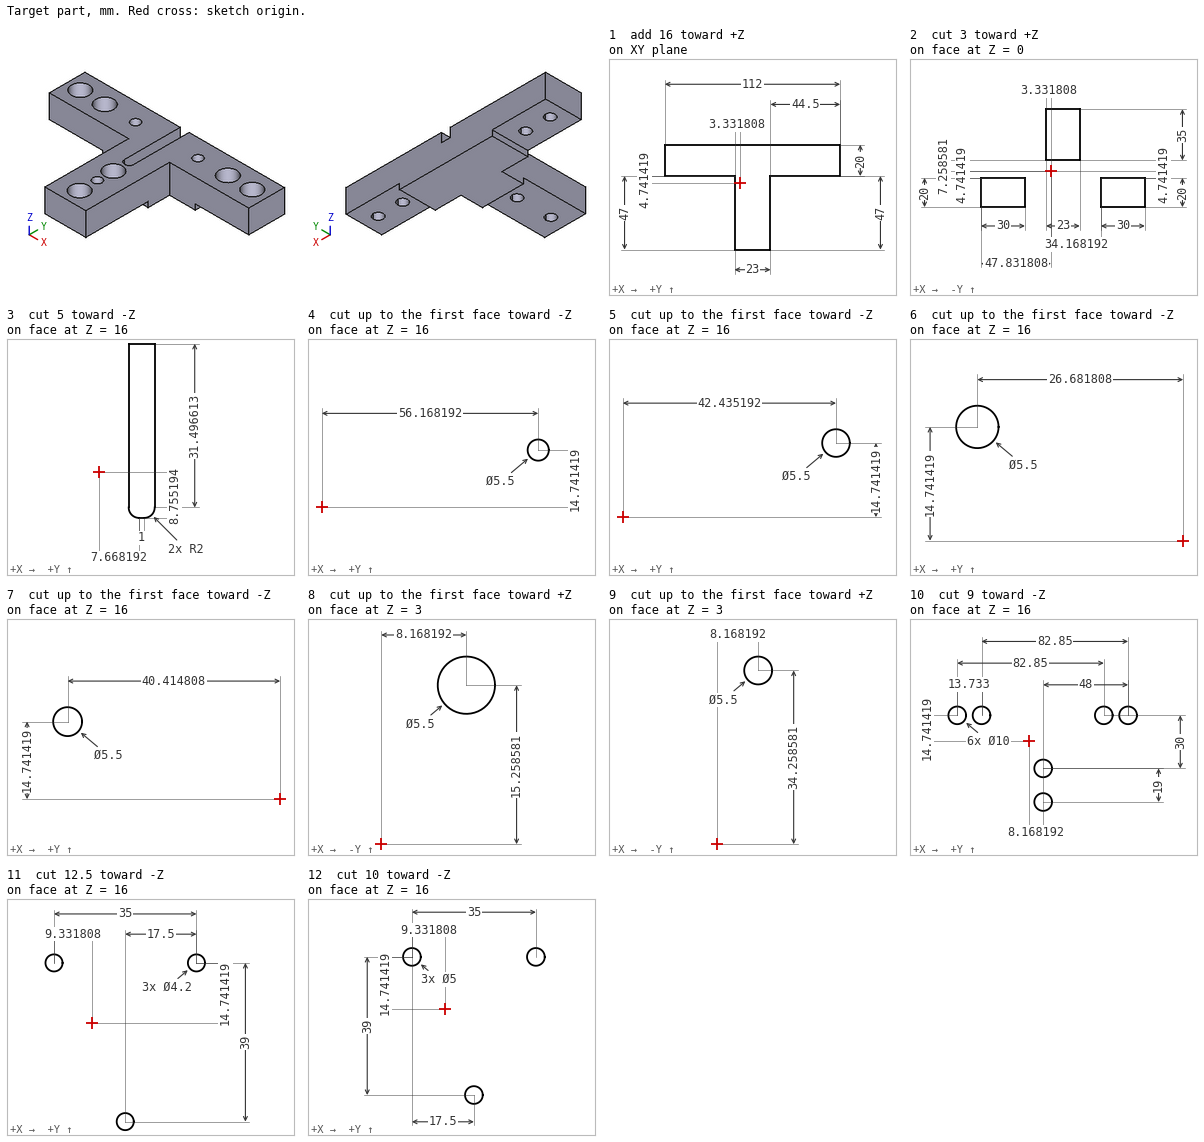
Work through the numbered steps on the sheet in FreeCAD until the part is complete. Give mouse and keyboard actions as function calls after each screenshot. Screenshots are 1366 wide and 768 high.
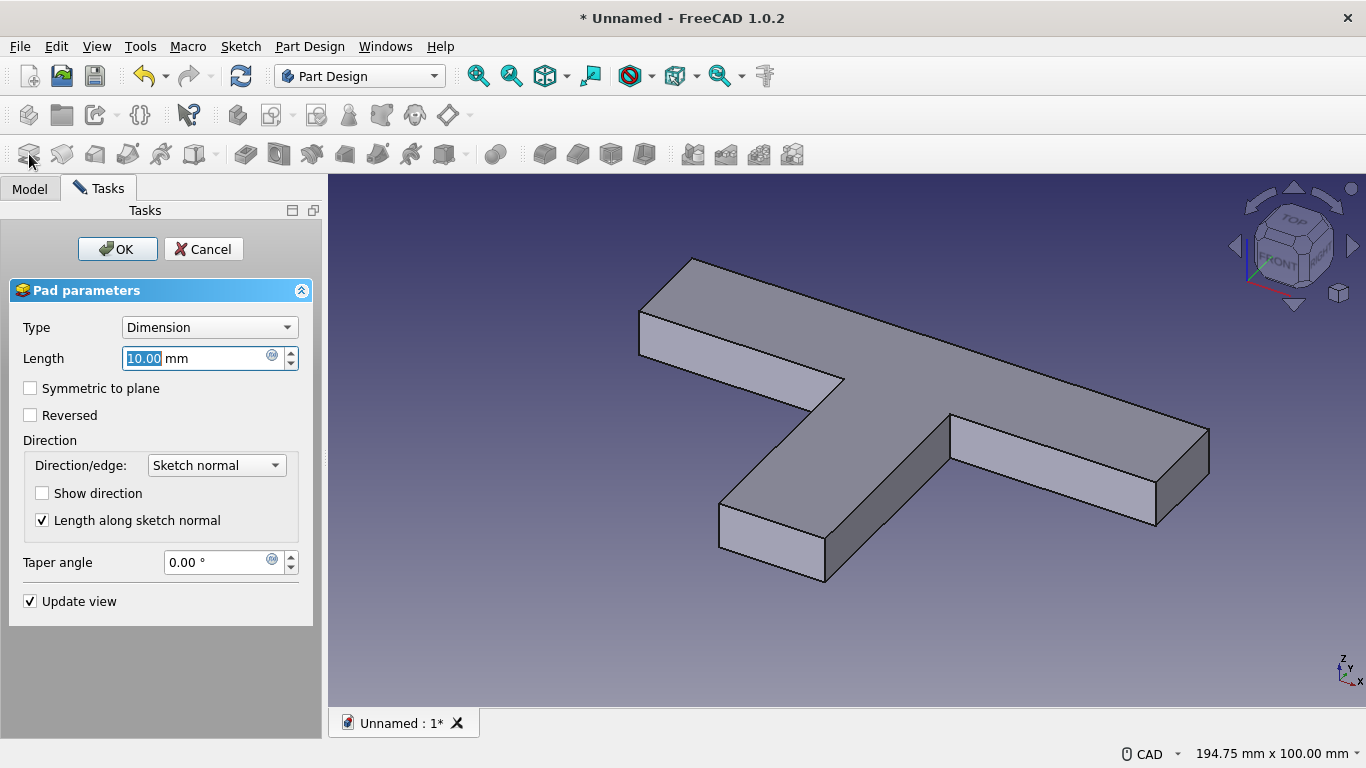
text(16)
key(Tab)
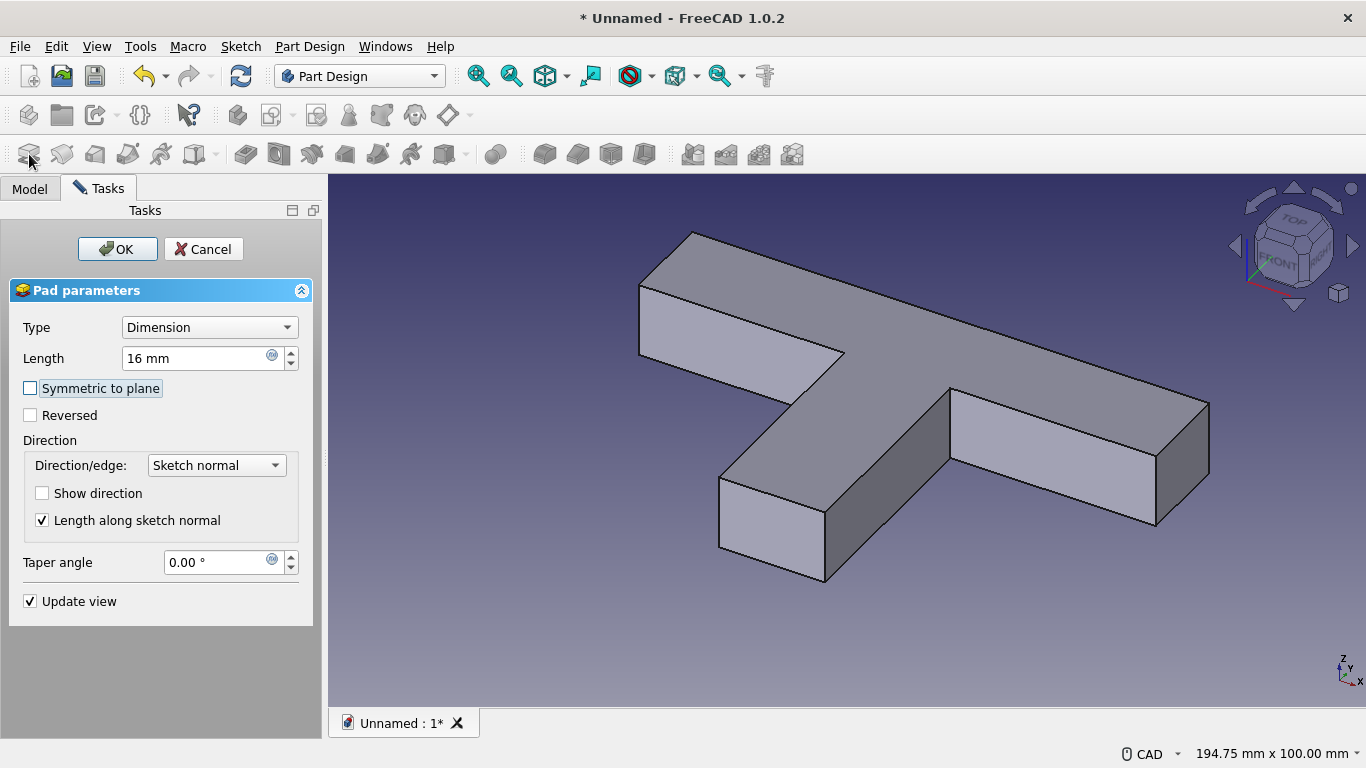
click(118, 249)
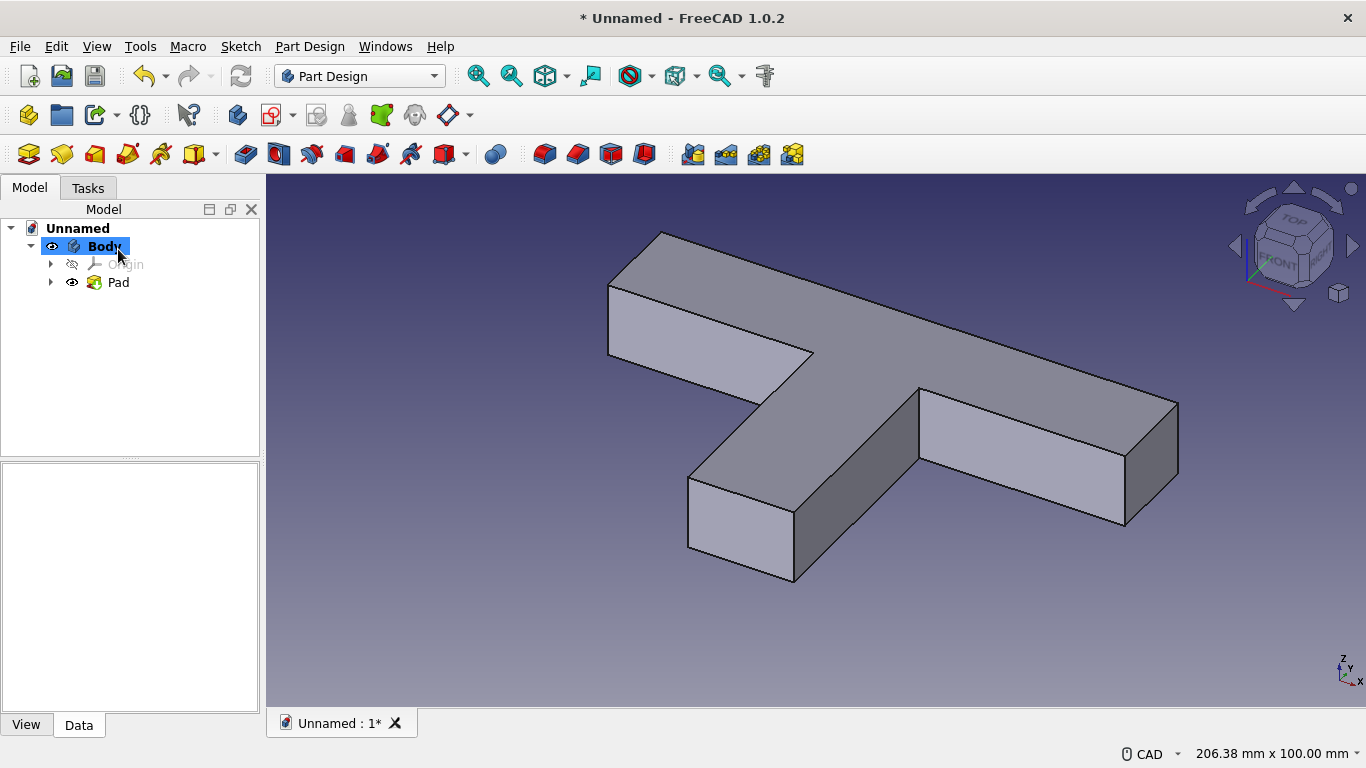
key(5)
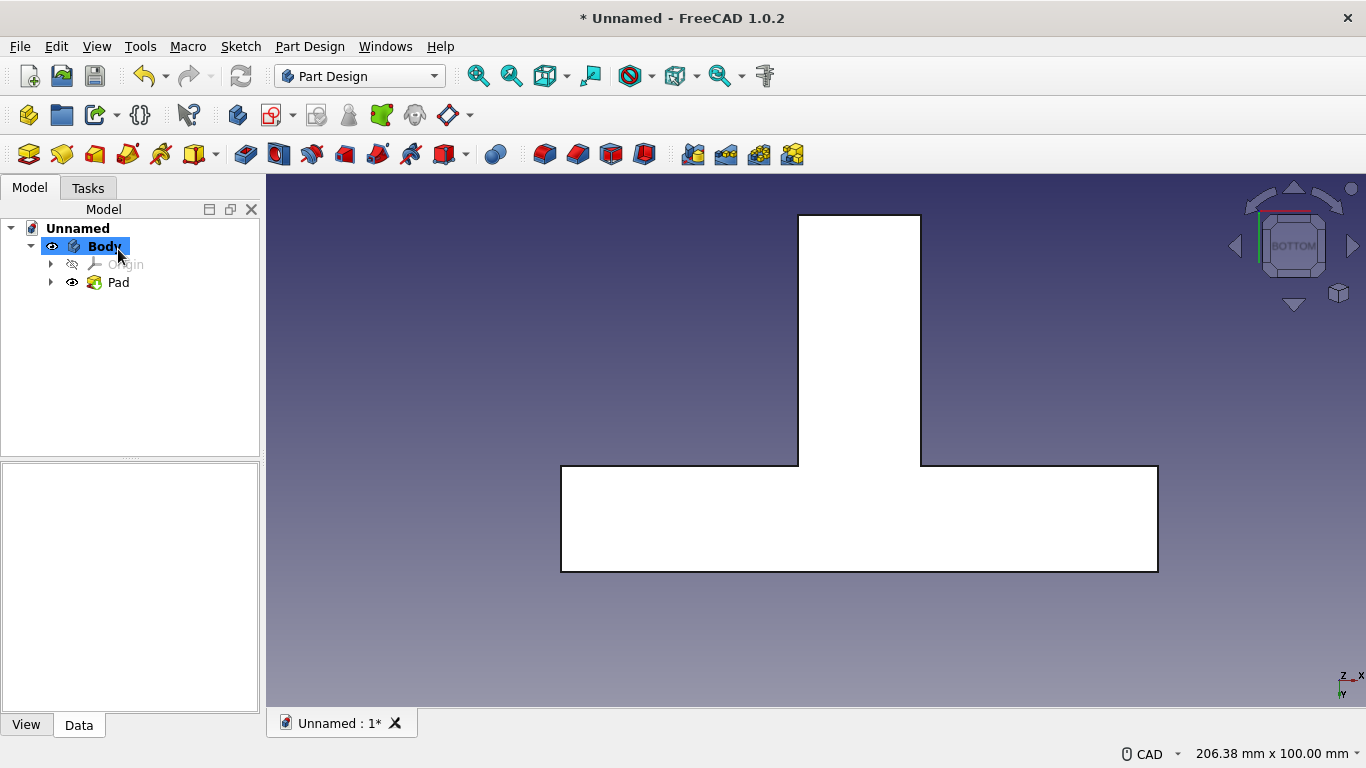
click(860, 495)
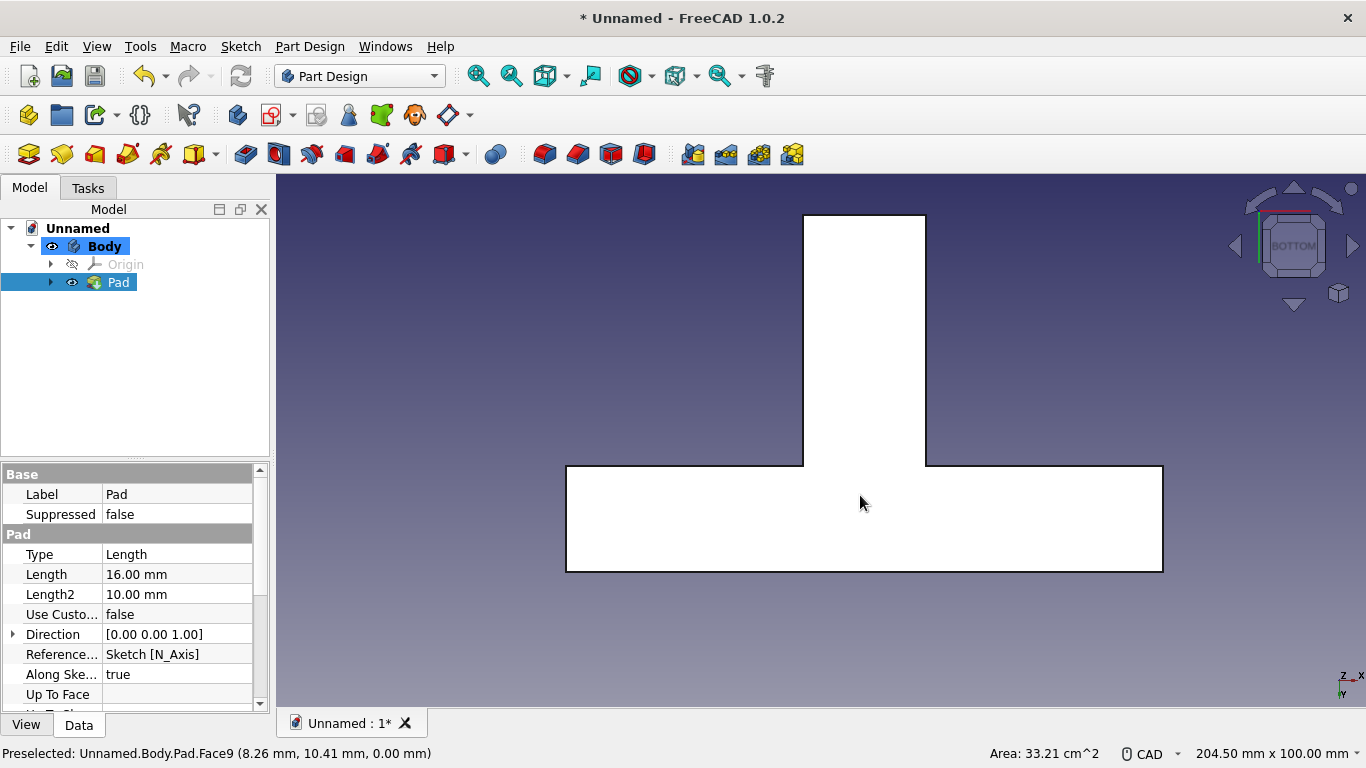
click(270, 116)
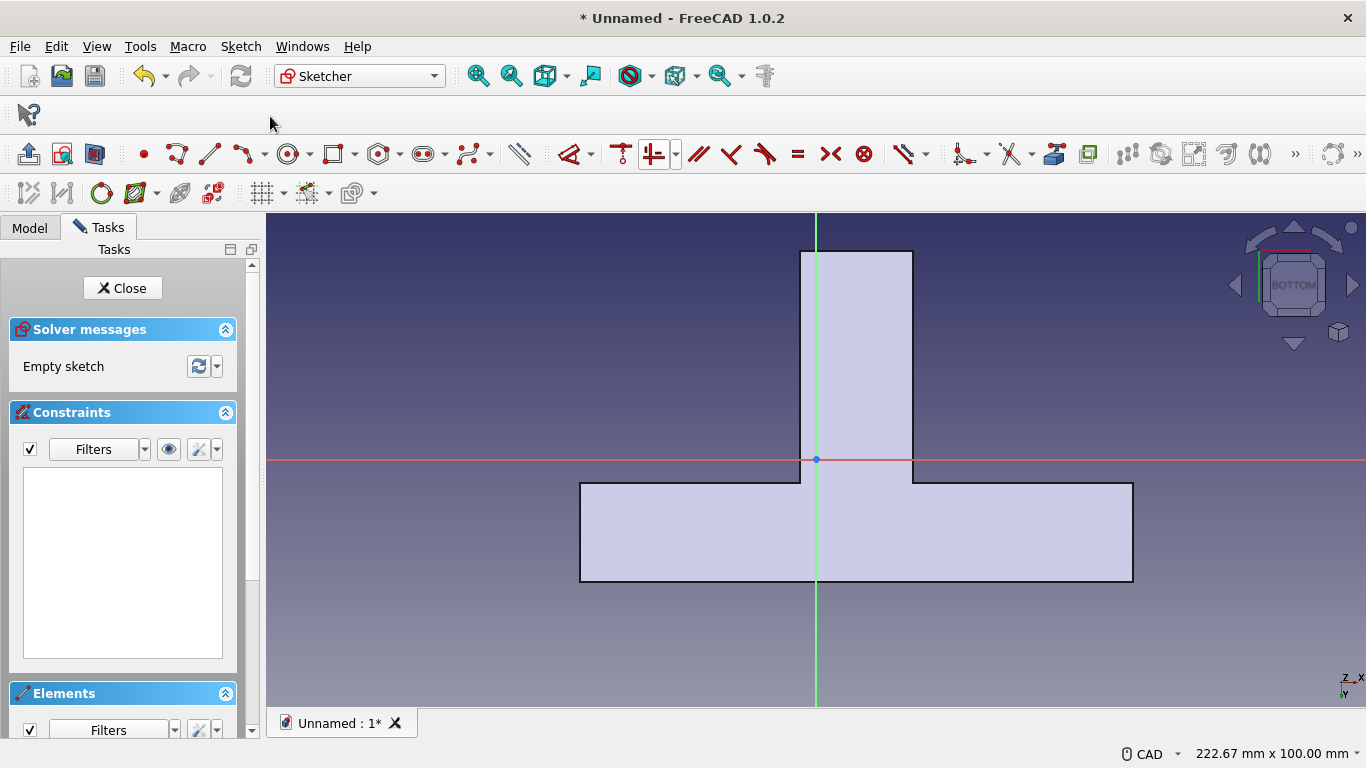
scroll(294, 655, down, 1)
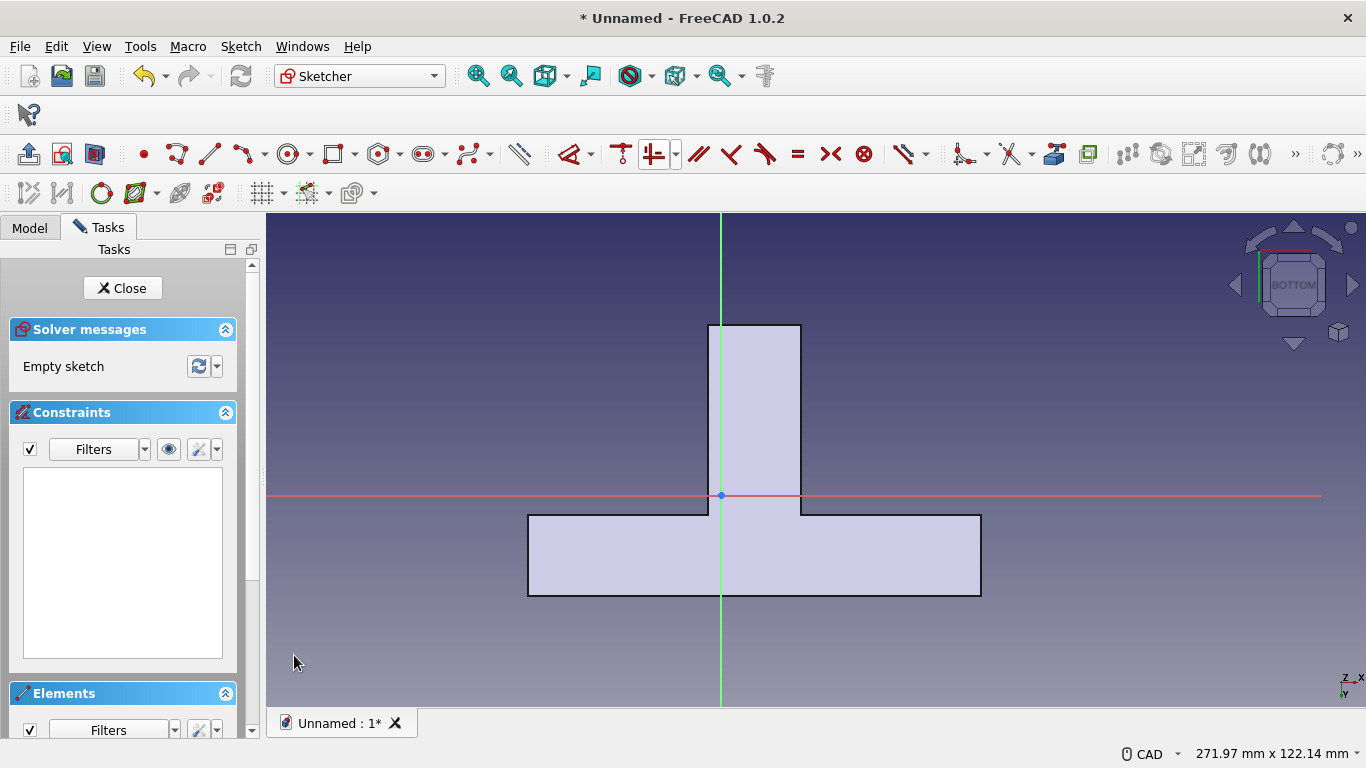
key(g)
key(r)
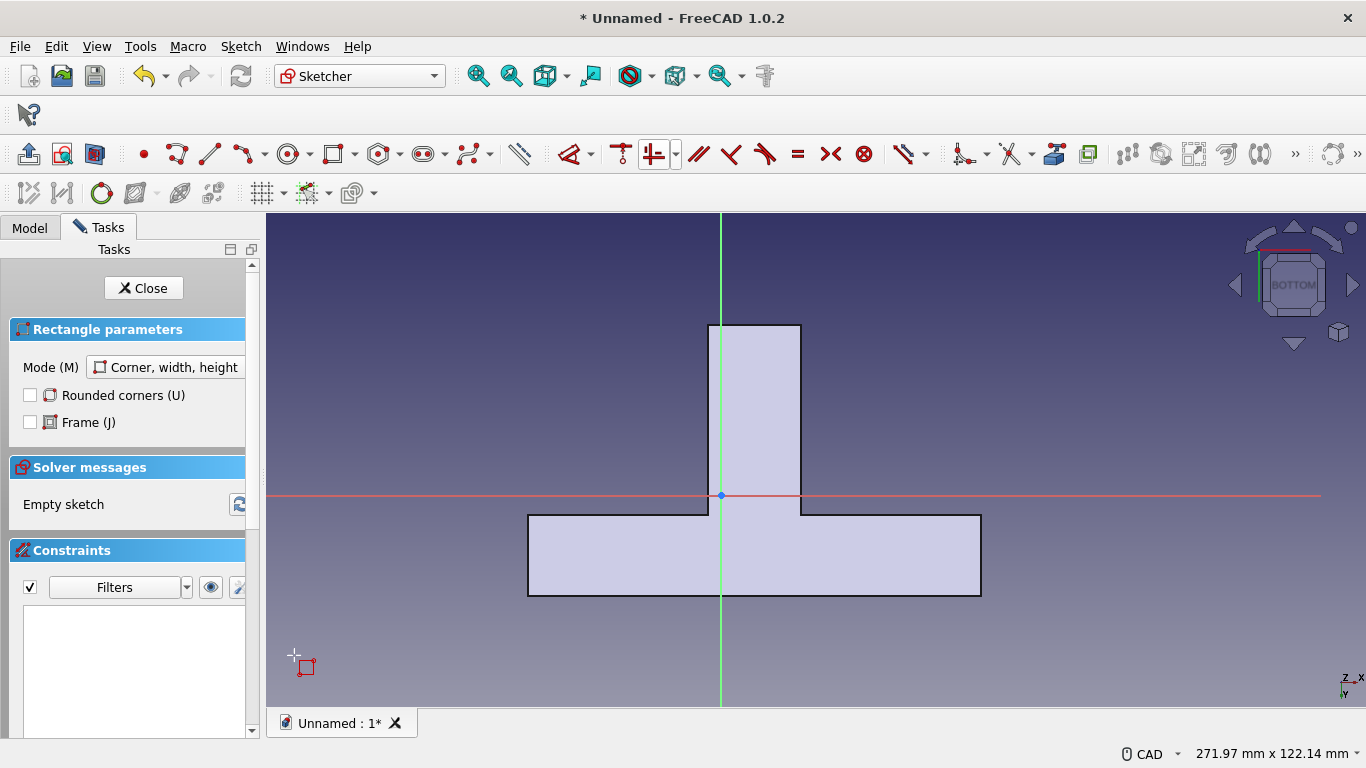
click(860, 515)
move(981, 596)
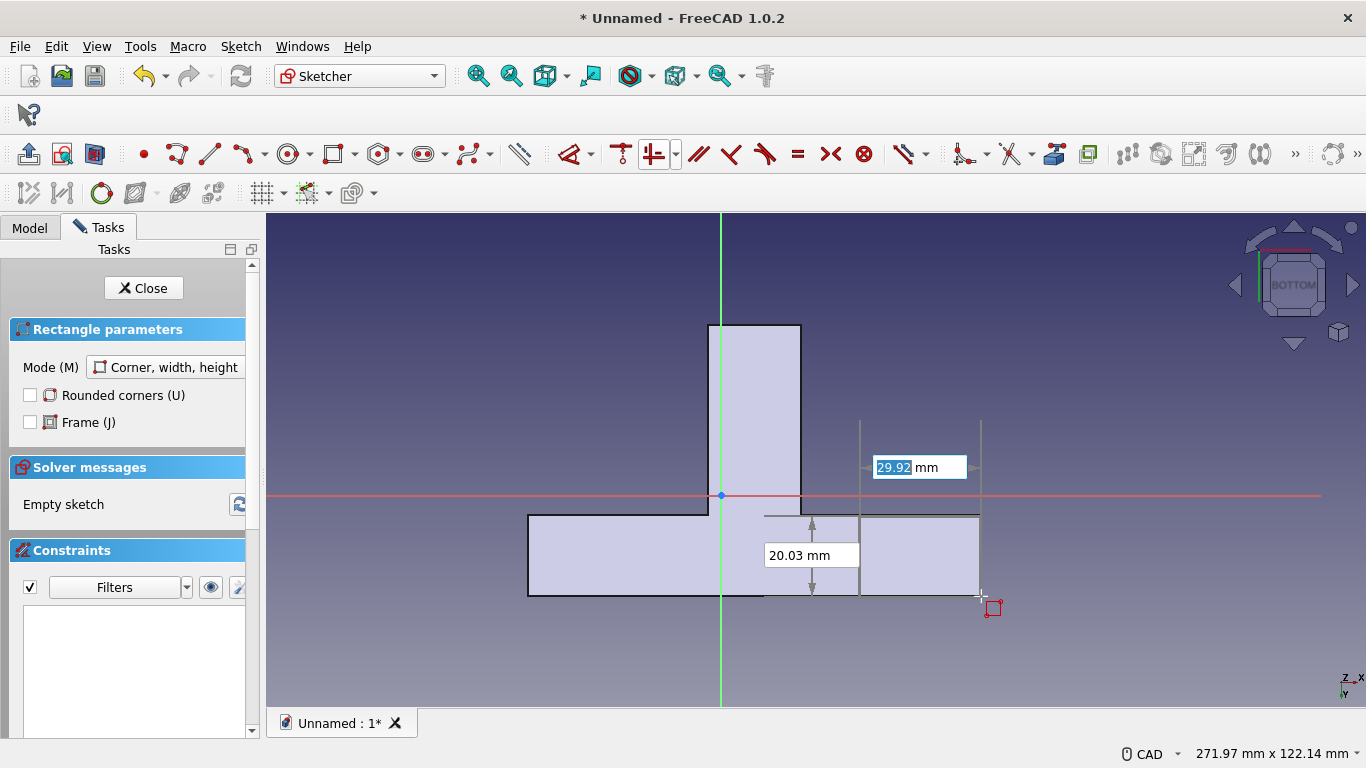
text(30)
key(Tab)
text(20)
key(Return)